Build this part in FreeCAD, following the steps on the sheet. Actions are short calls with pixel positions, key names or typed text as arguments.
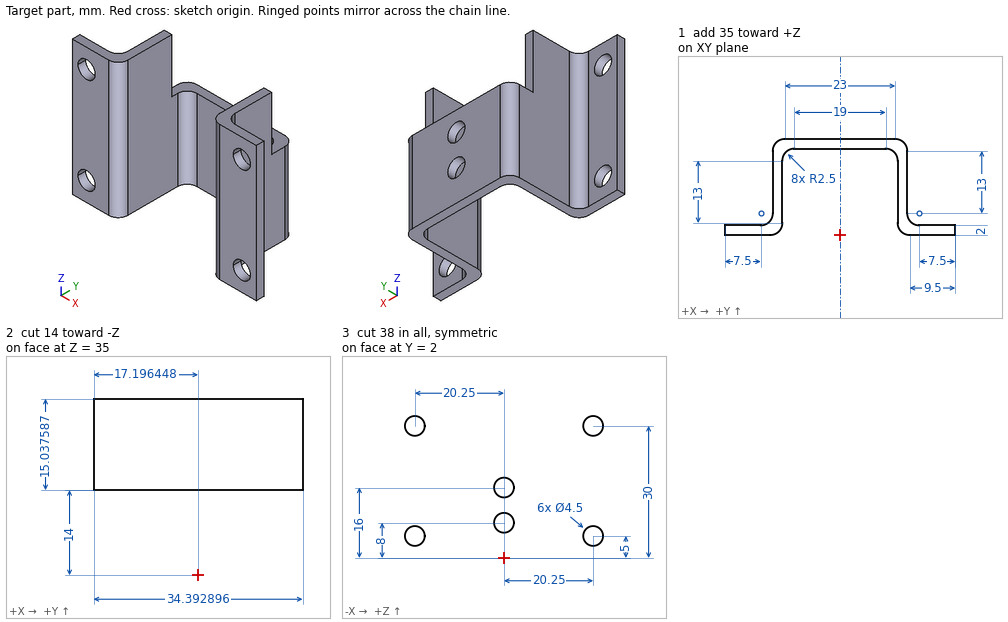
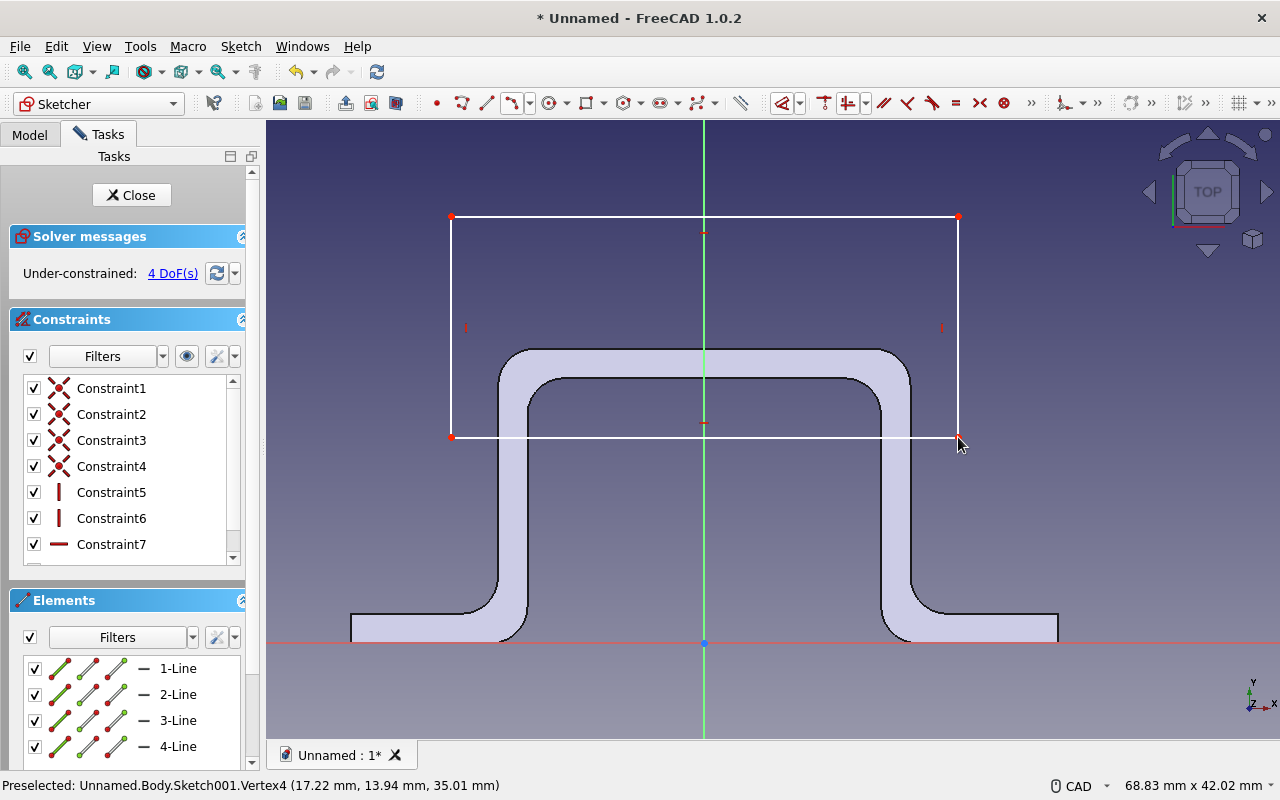
click(451, 438)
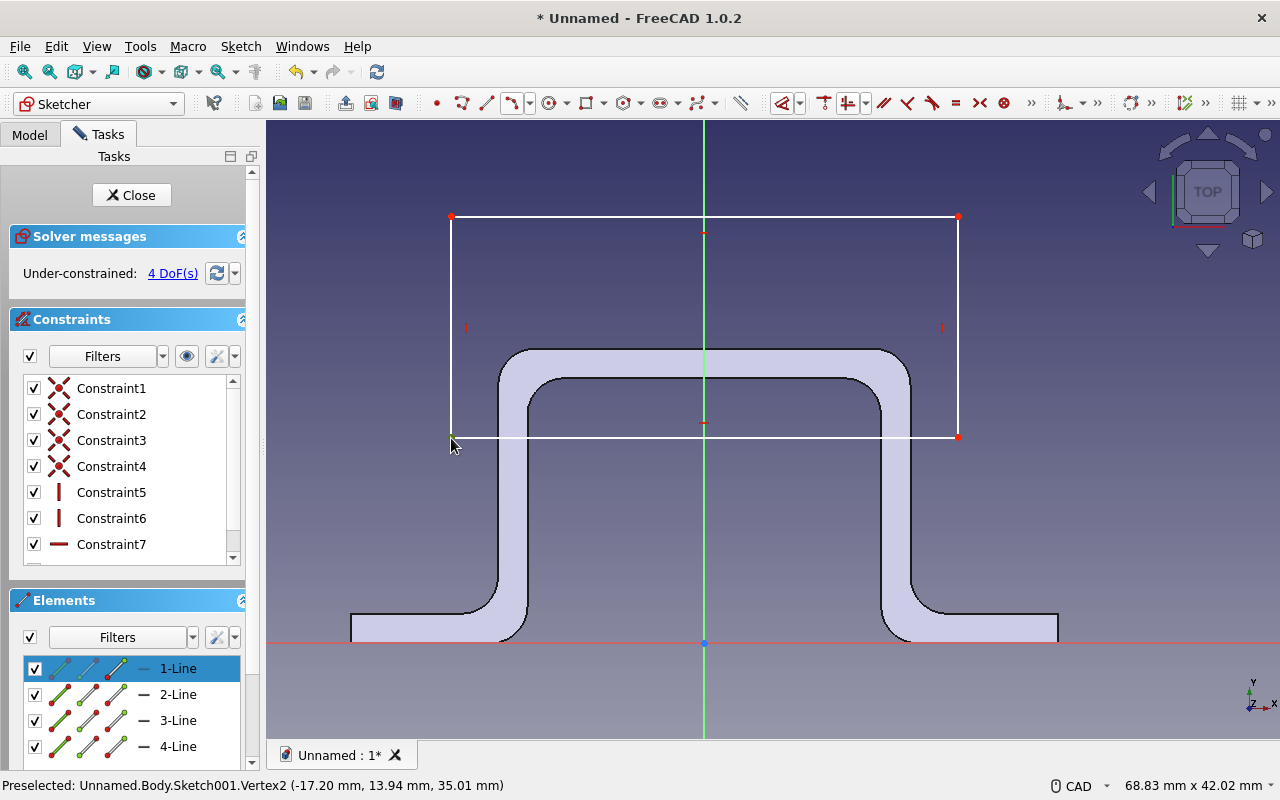
key(i)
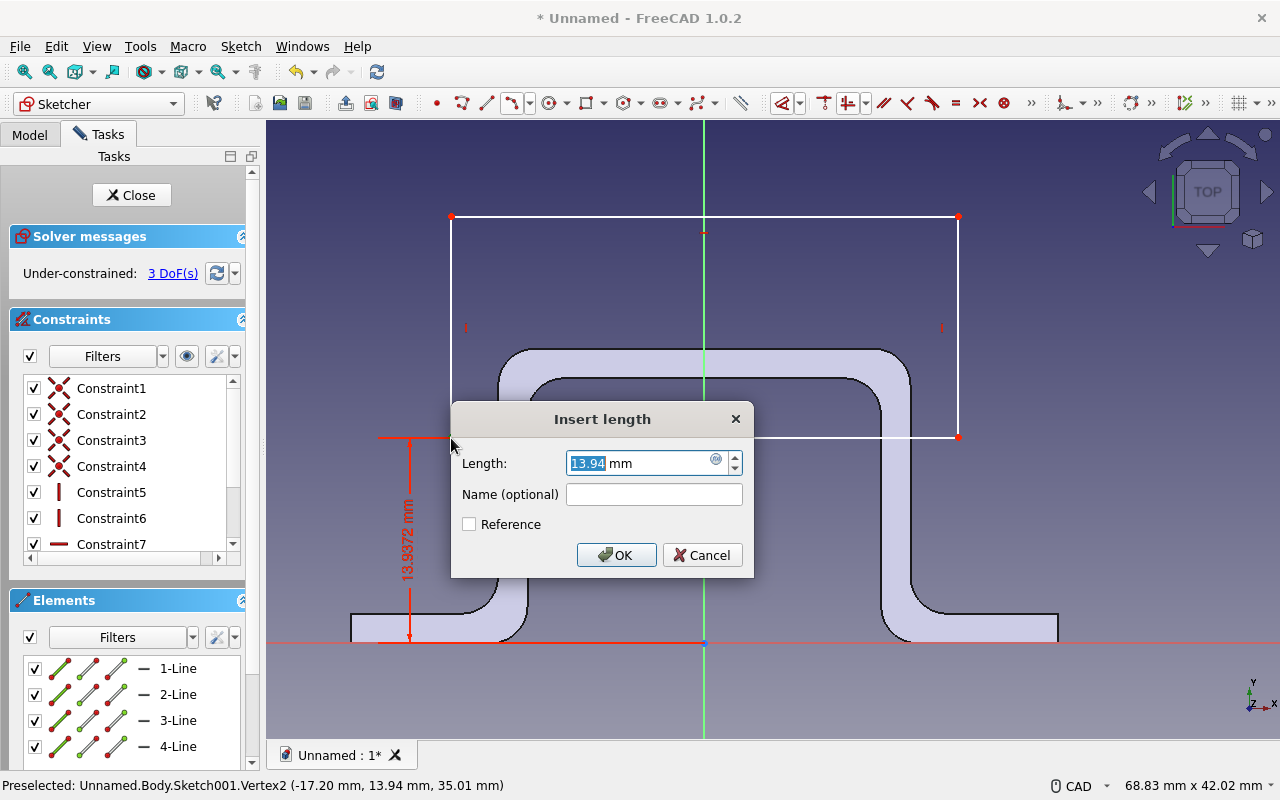
text(14)
key(Return)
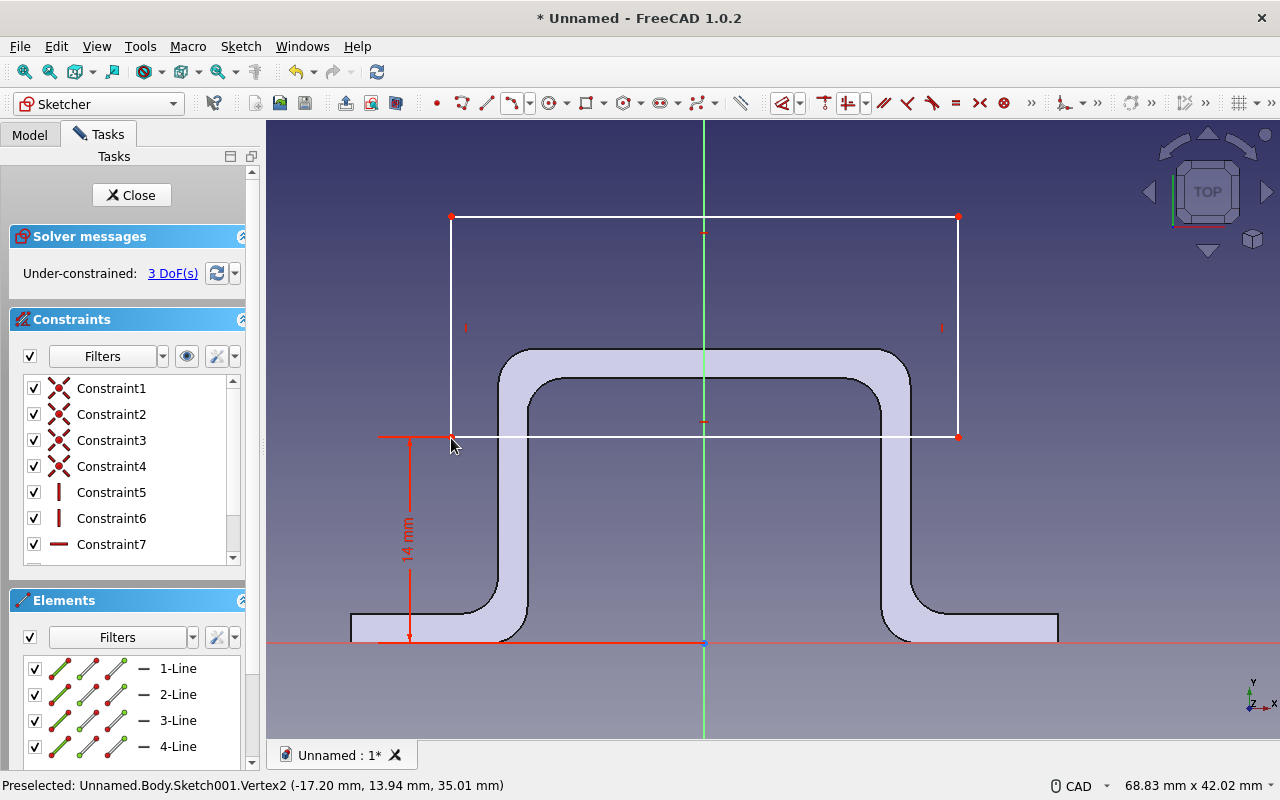
click(451, 283)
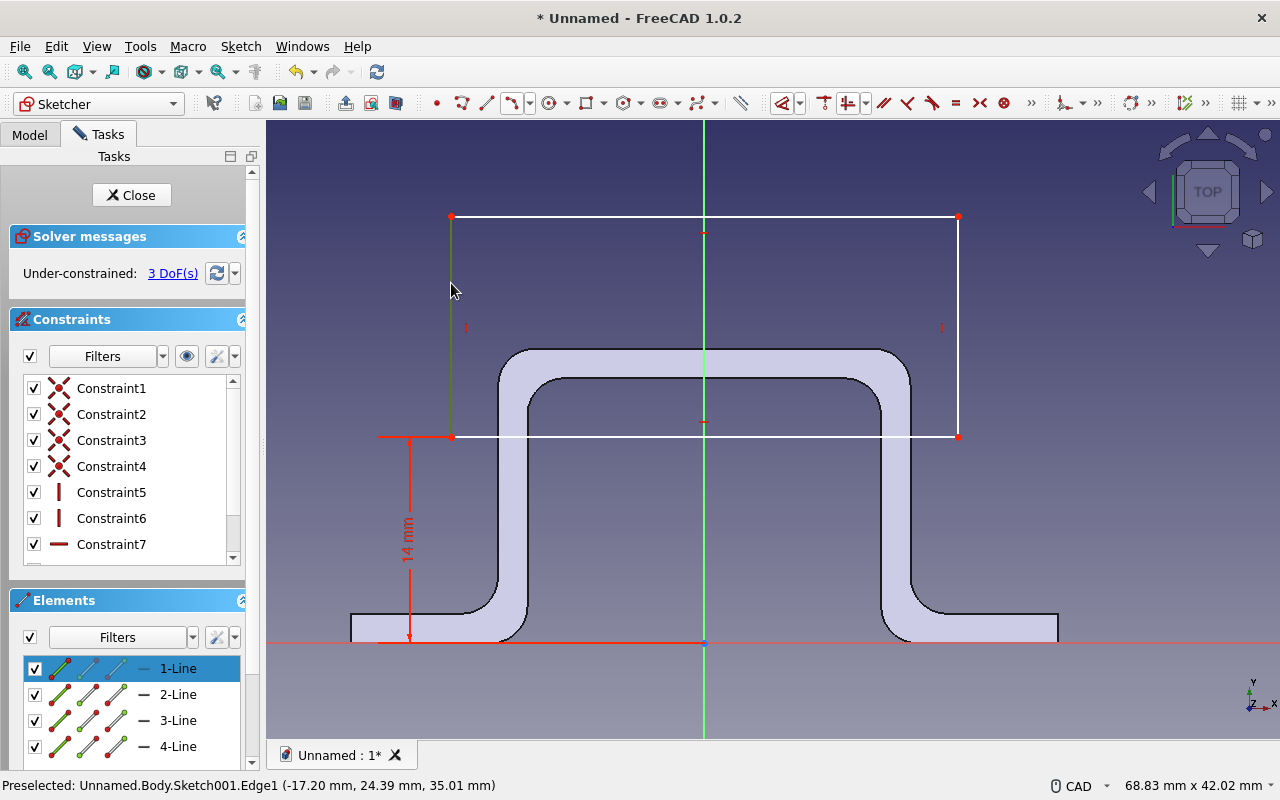
key(i)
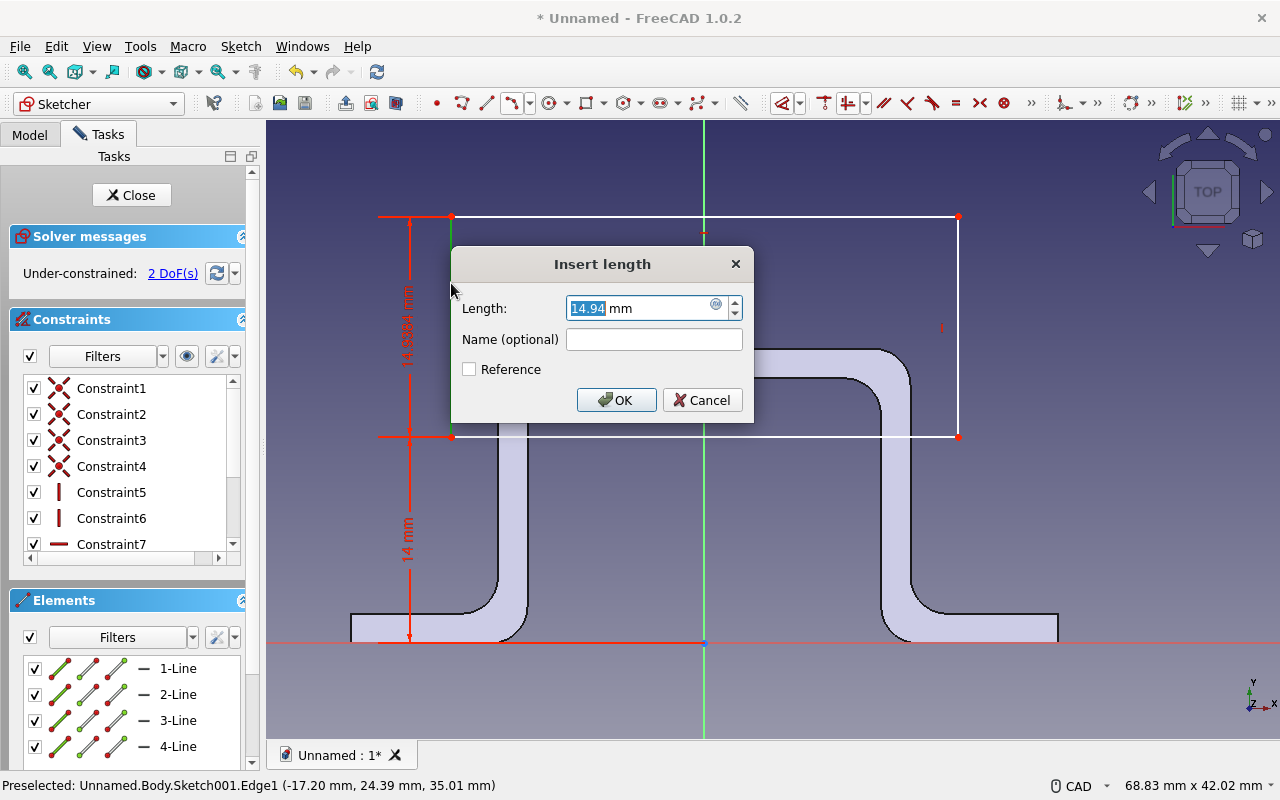
text(15.037587)
key(Return)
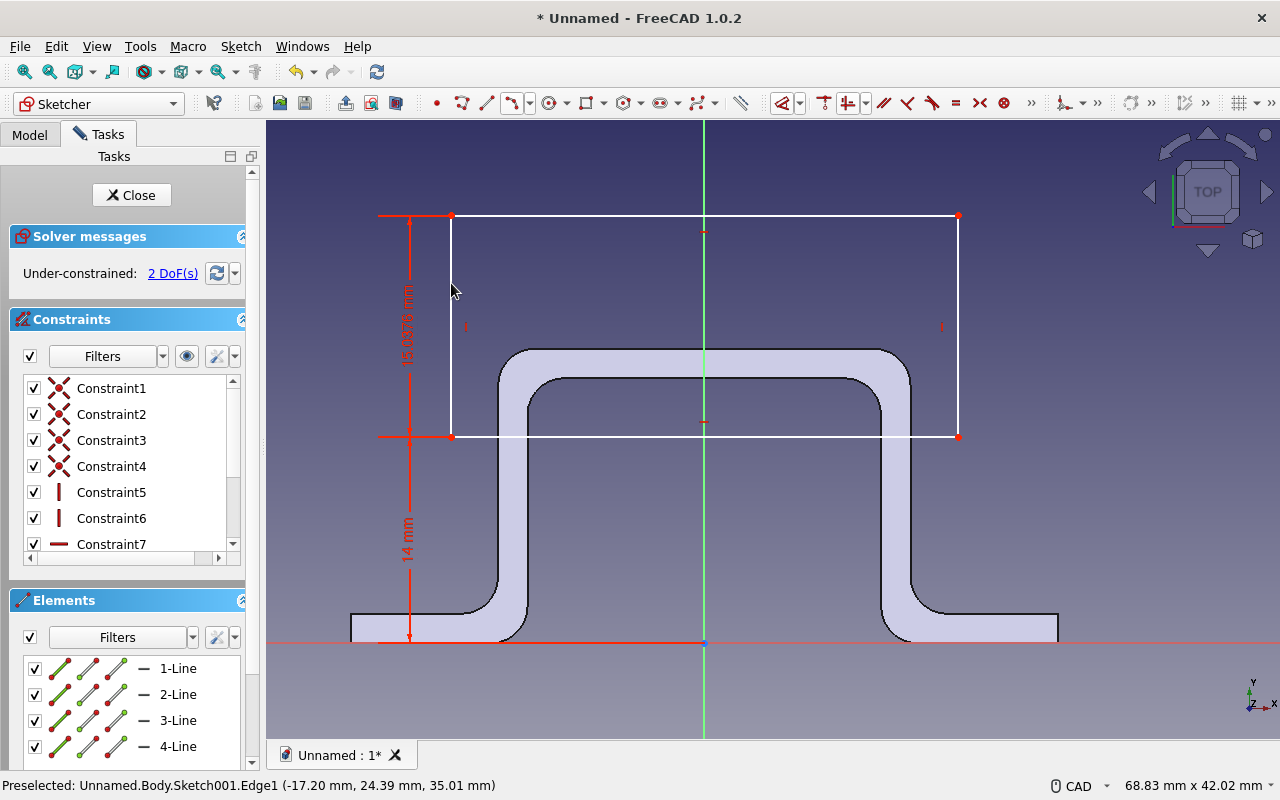
click(603, 437)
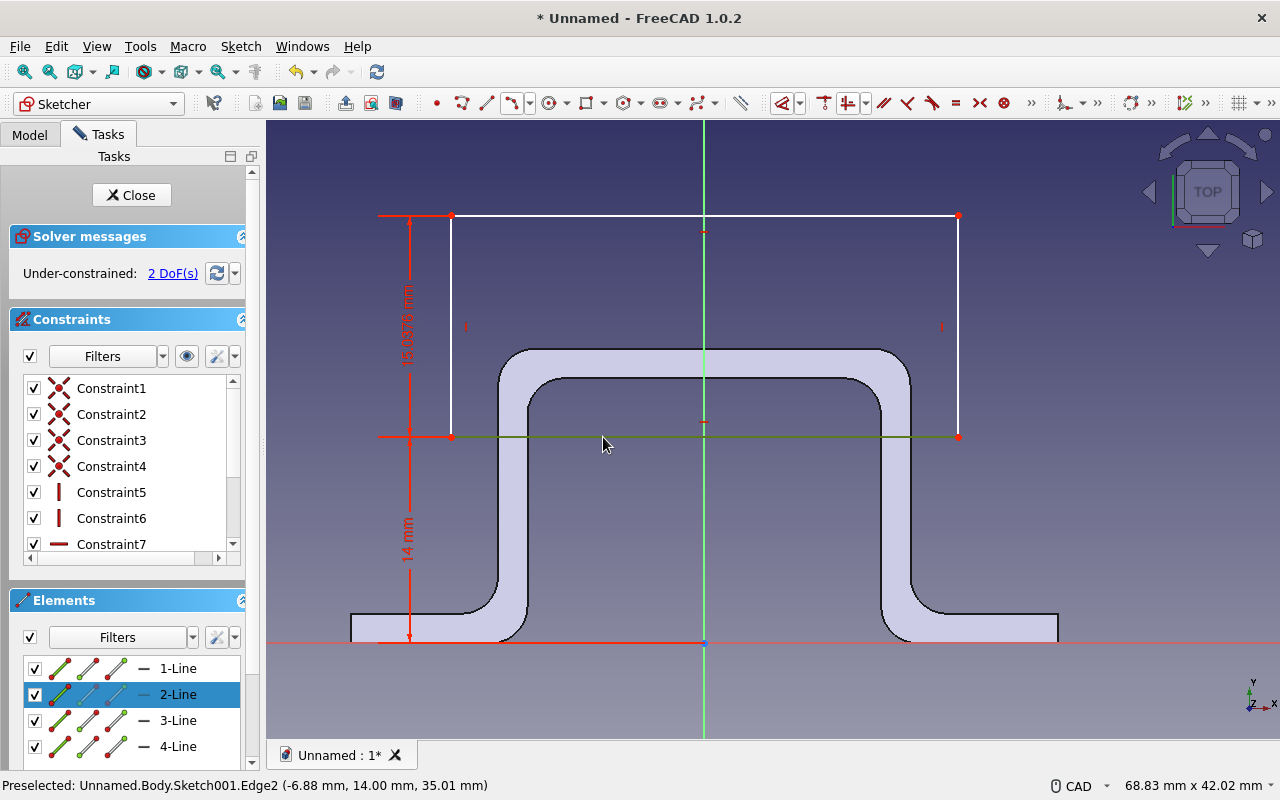
click(800, 104)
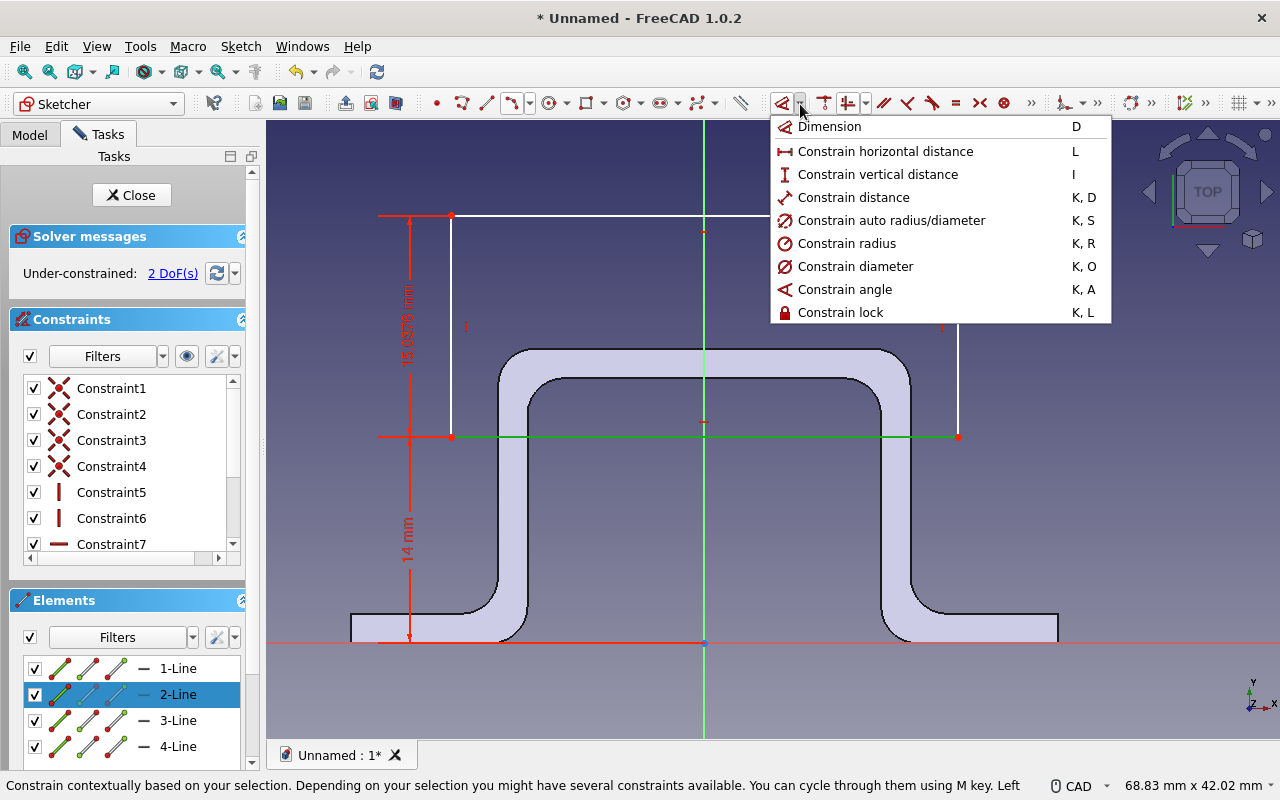
click(941, 152)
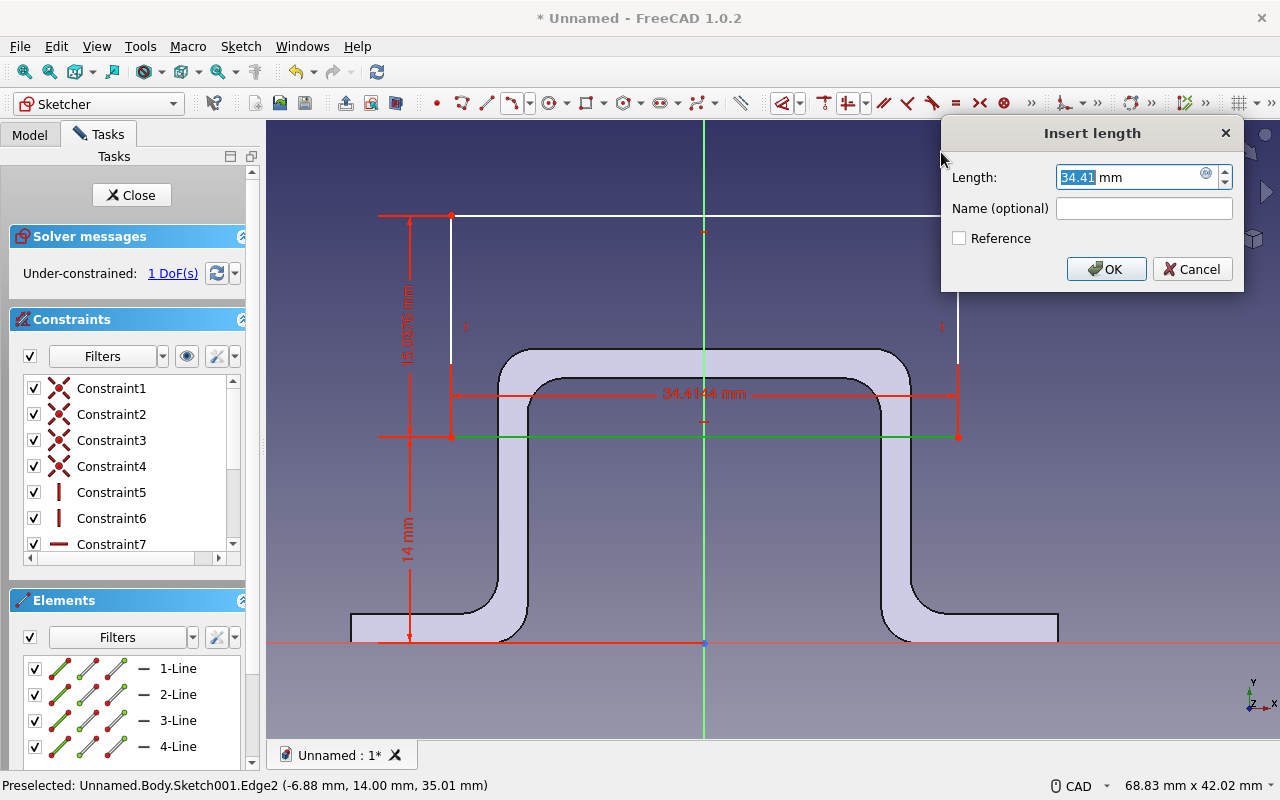
text(34.392896)
key(Return)